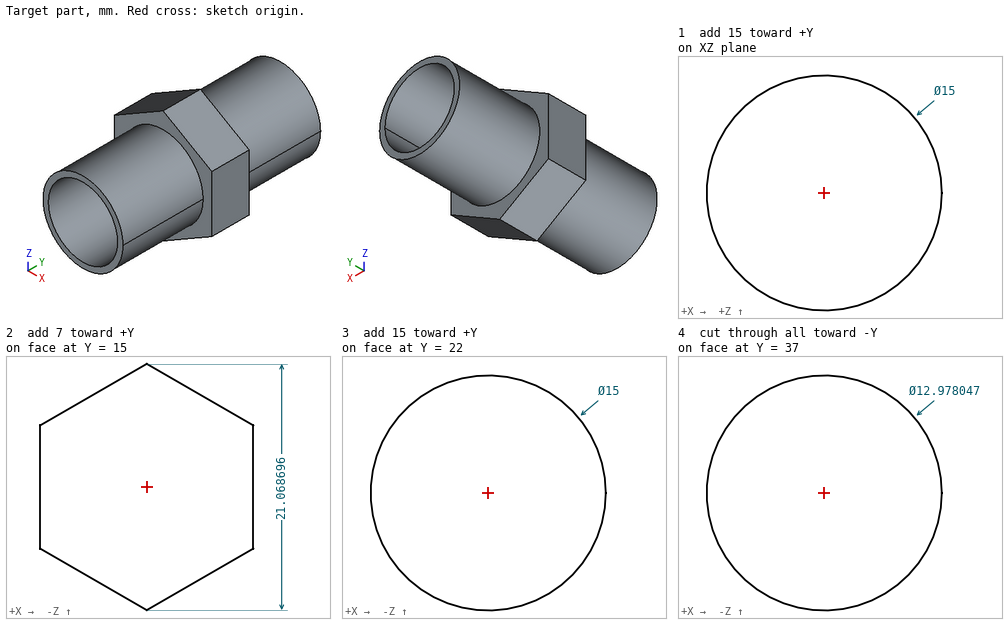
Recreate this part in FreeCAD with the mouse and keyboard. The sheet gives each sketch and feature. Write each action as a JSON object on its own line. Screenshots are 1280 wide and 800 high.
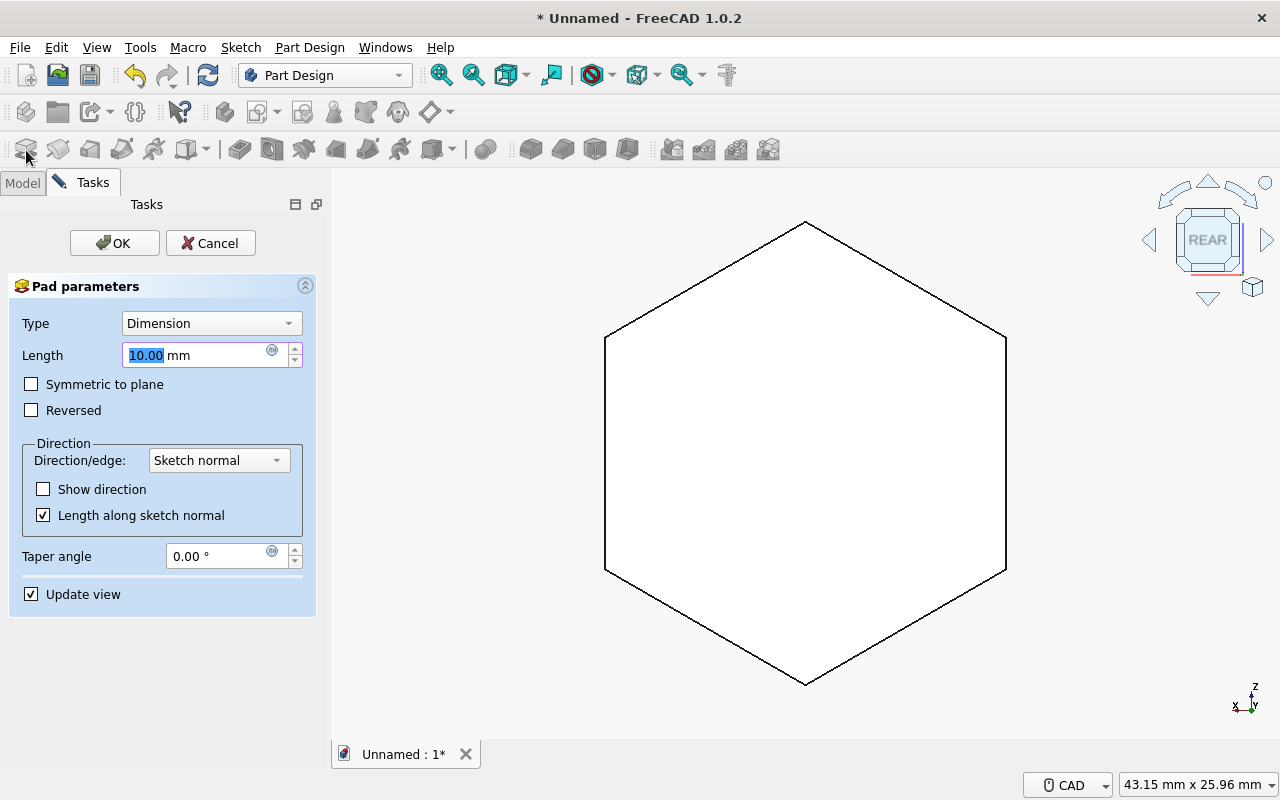
{"action": "type", "text": "7"}
{"action": "key", "text": "Tab"}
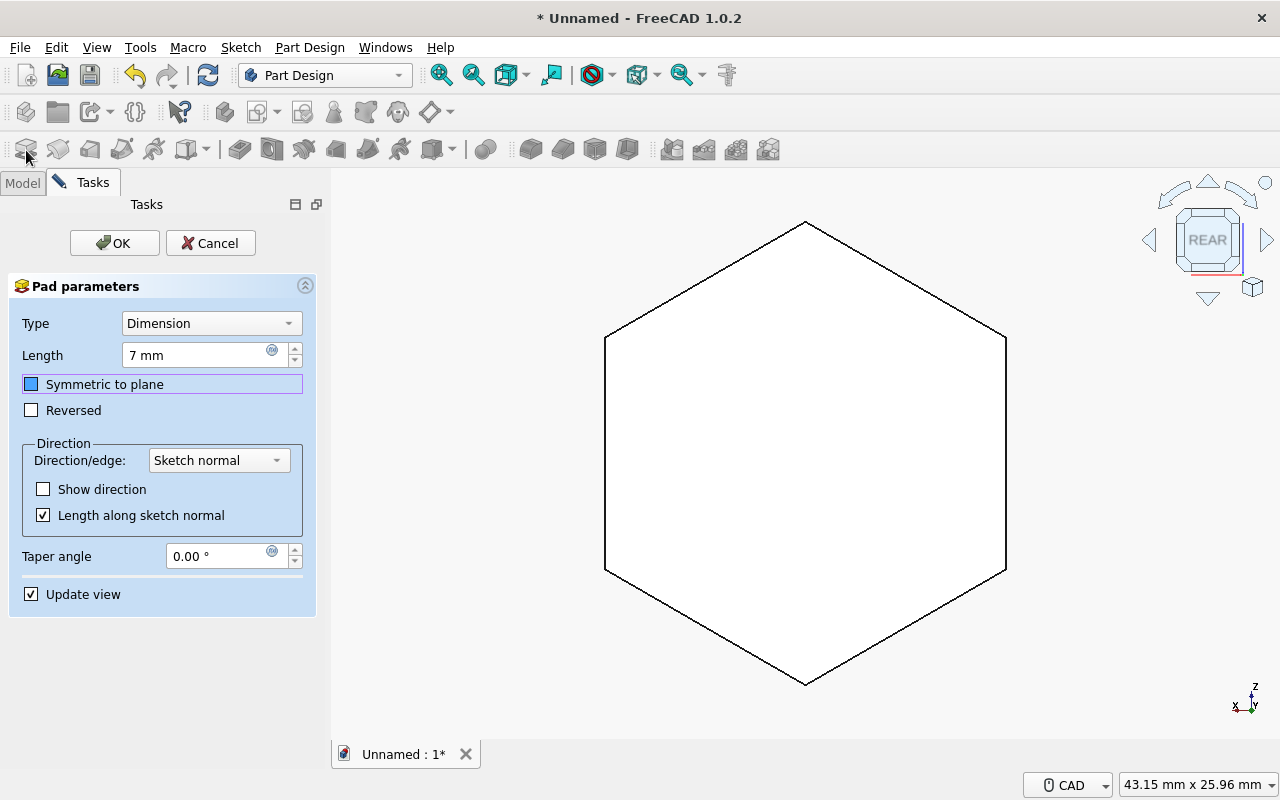
{"action": "left_click", "coordinate": [115, 243]}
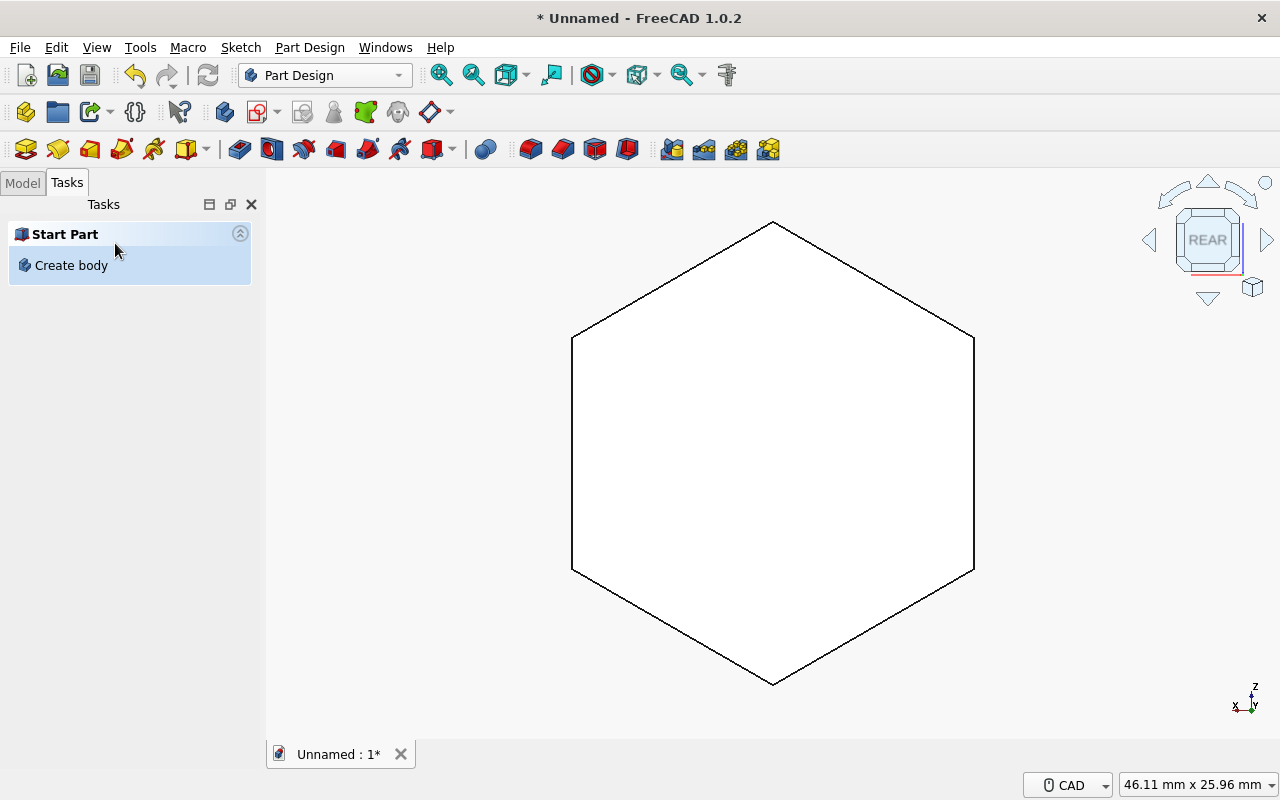
{"action": "left_click", "coordinate": [773, 453]}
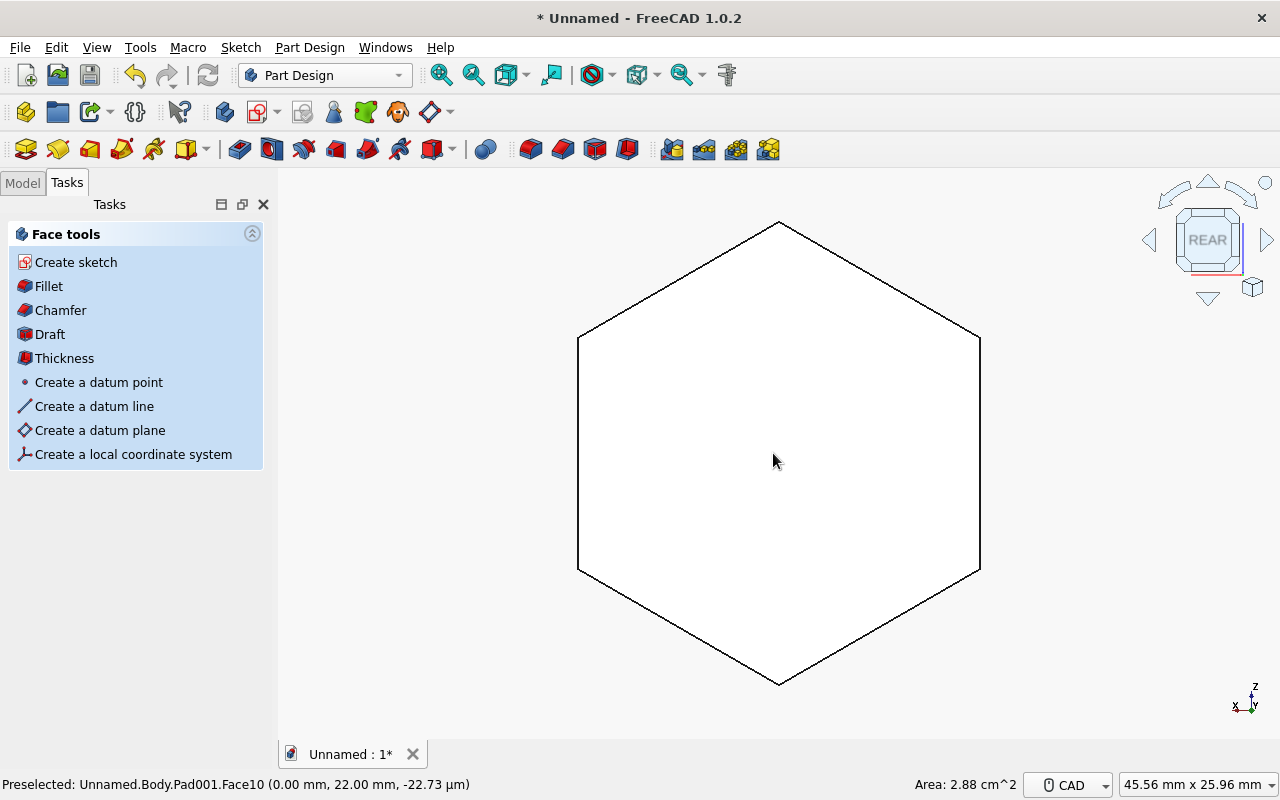
{"action": "left_click", "coordinate": [258, 112]}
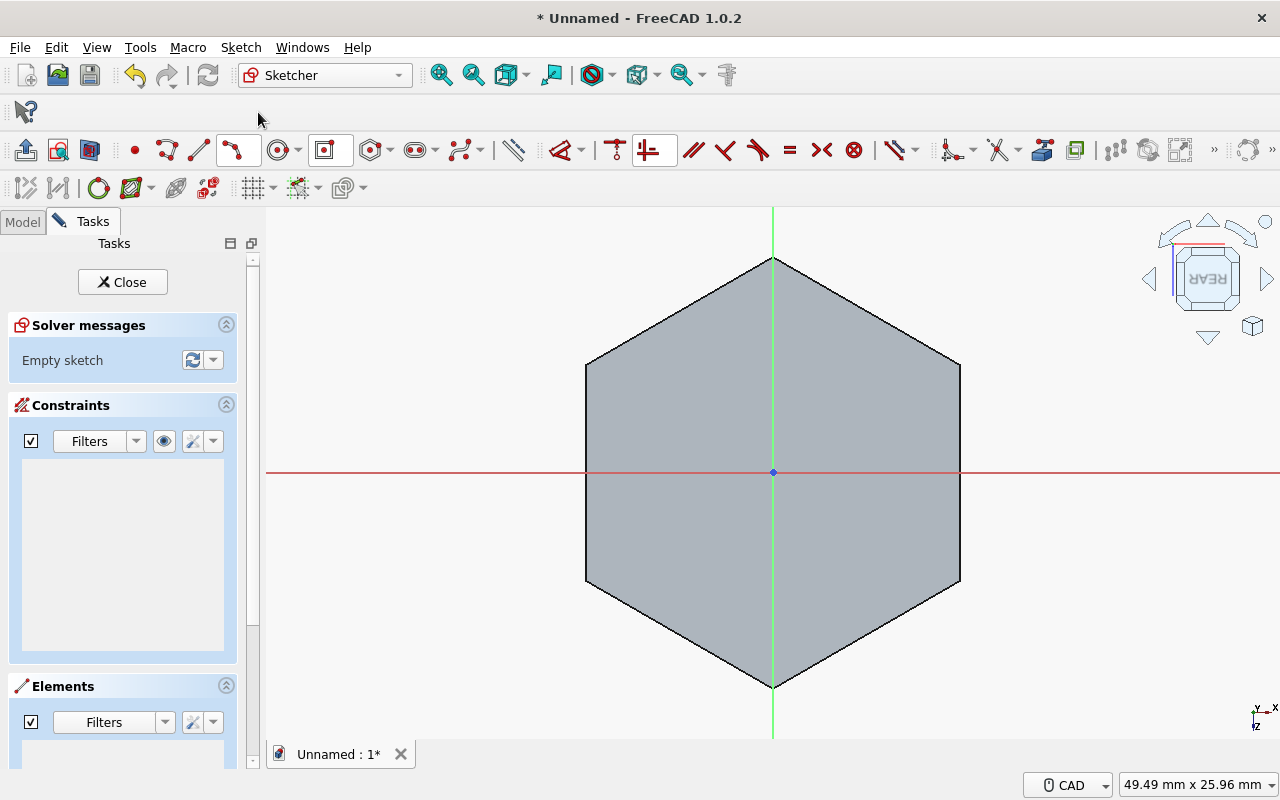
{"action": "left_click", "coordinate": [278, 150]}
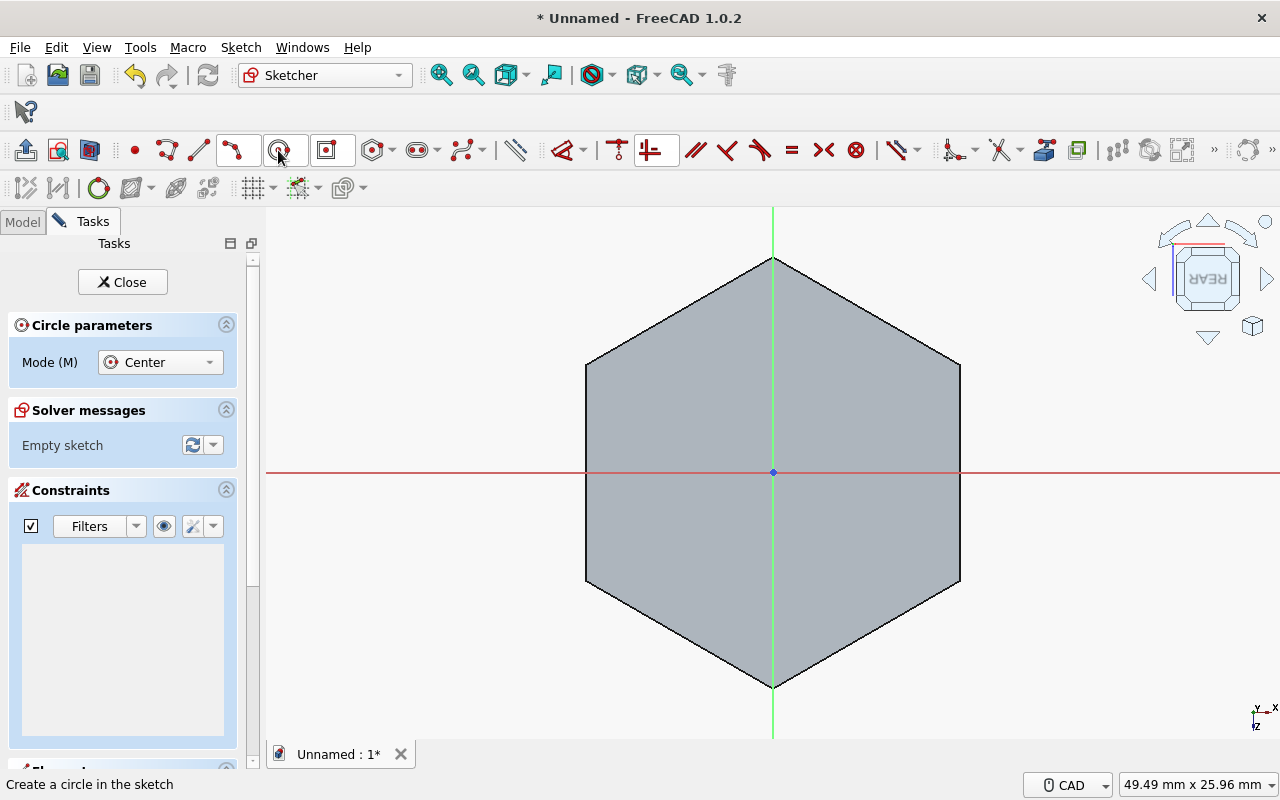
{"action": "left_click", "coordinate": [773, 473]}
{"action": "mouse_move", "coordinate": [882, 364]}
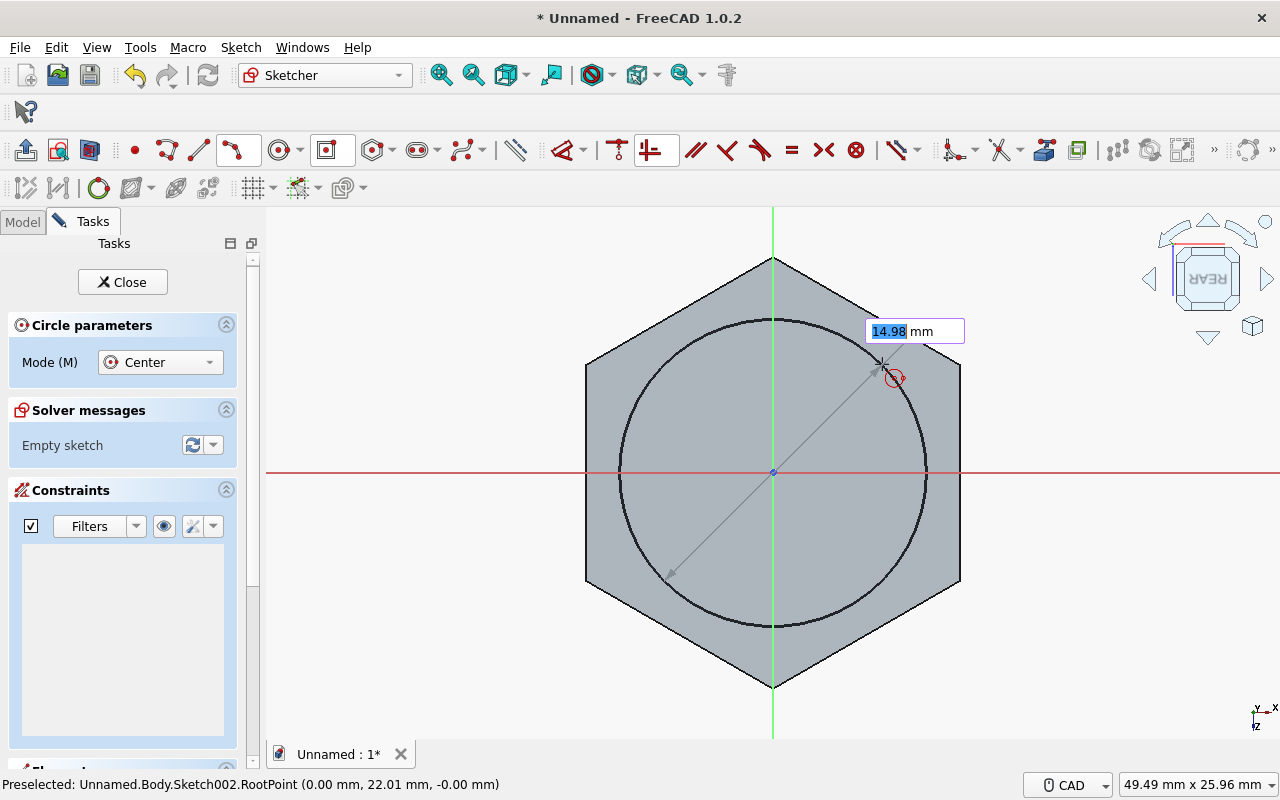
{"action": "type", "text": "15"}
{"action": "key", "text": "Return"}
{"action": "key", "text": "Escape"}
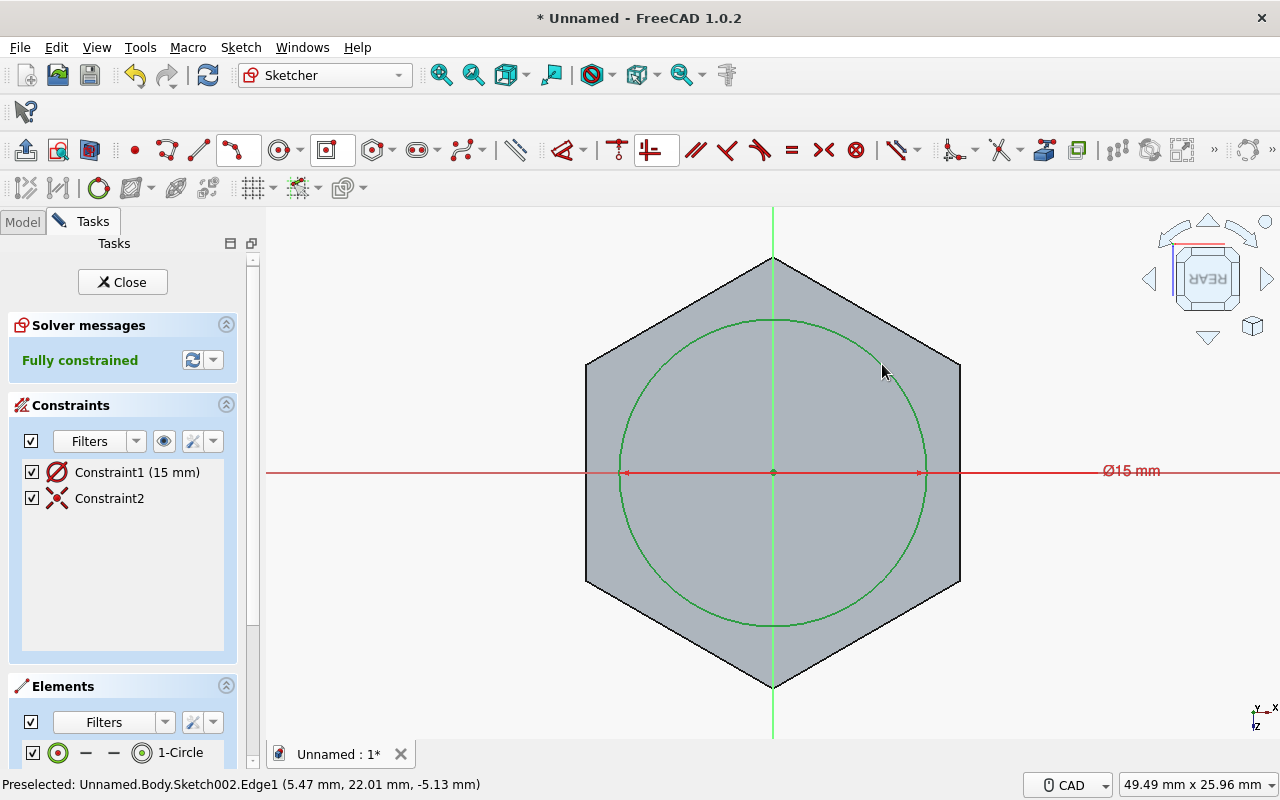
{"action": "left_click", "coordinate": [123, 282]}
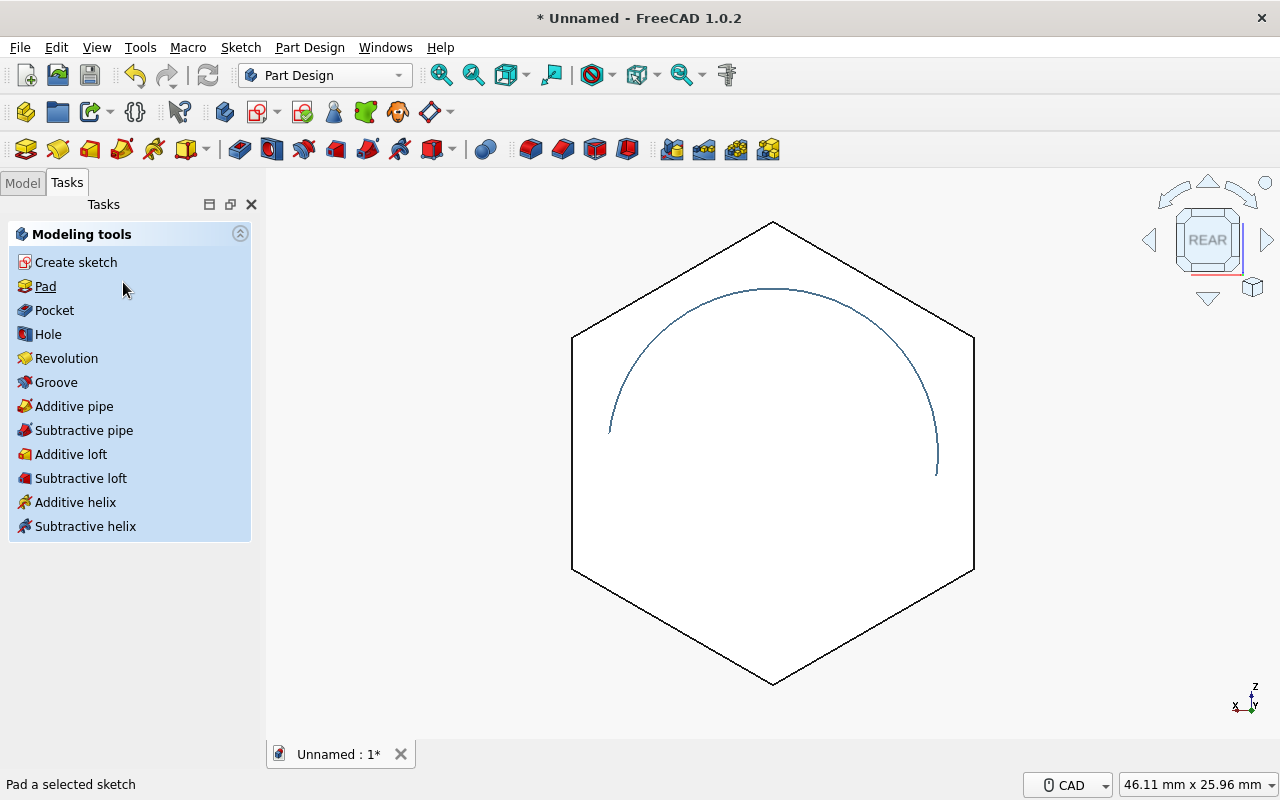
{"action": "left_click", "coordinate": [26, 150]}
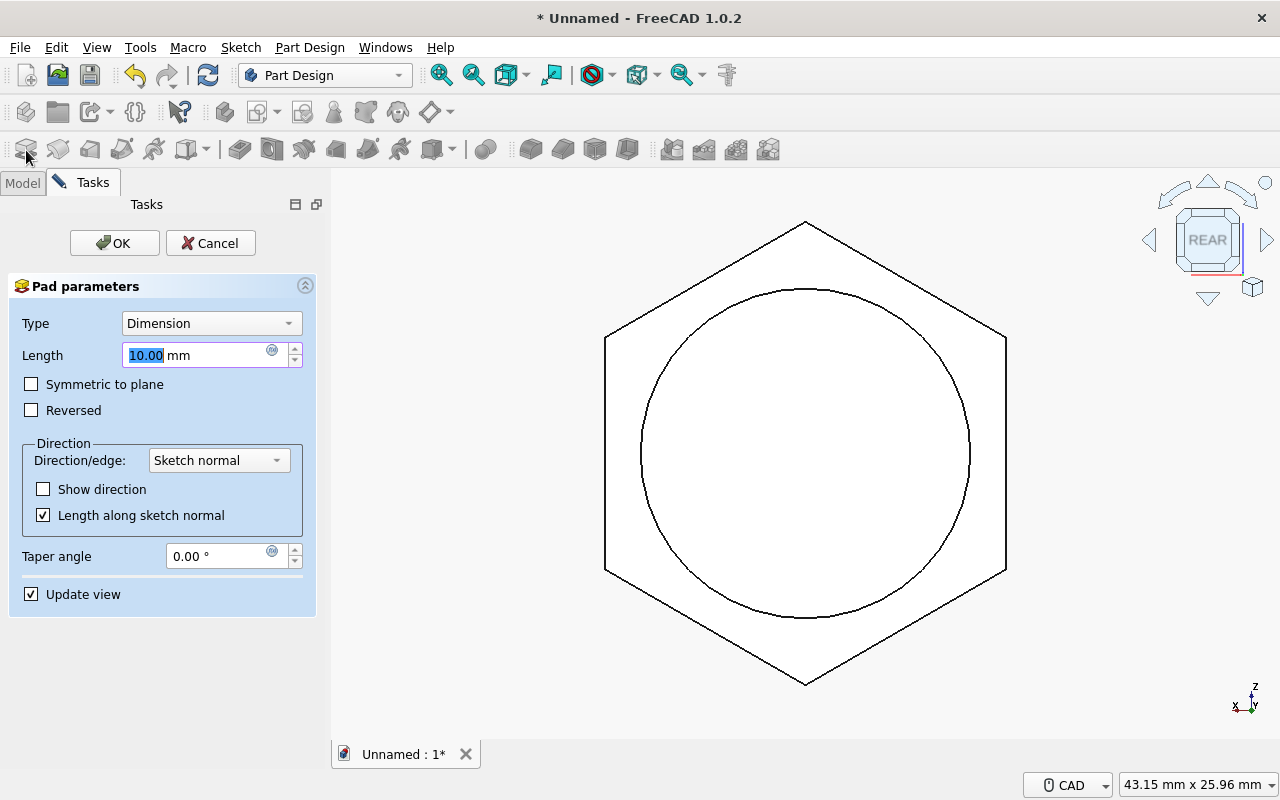
{"action": "type", "text": "15"}
{"action": "key", "text": "Tab"}